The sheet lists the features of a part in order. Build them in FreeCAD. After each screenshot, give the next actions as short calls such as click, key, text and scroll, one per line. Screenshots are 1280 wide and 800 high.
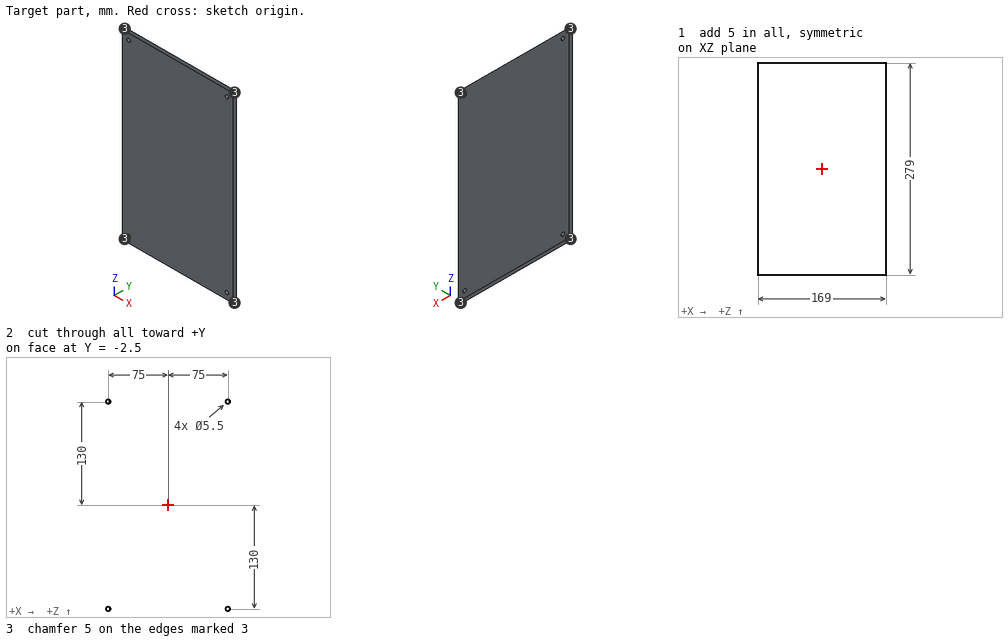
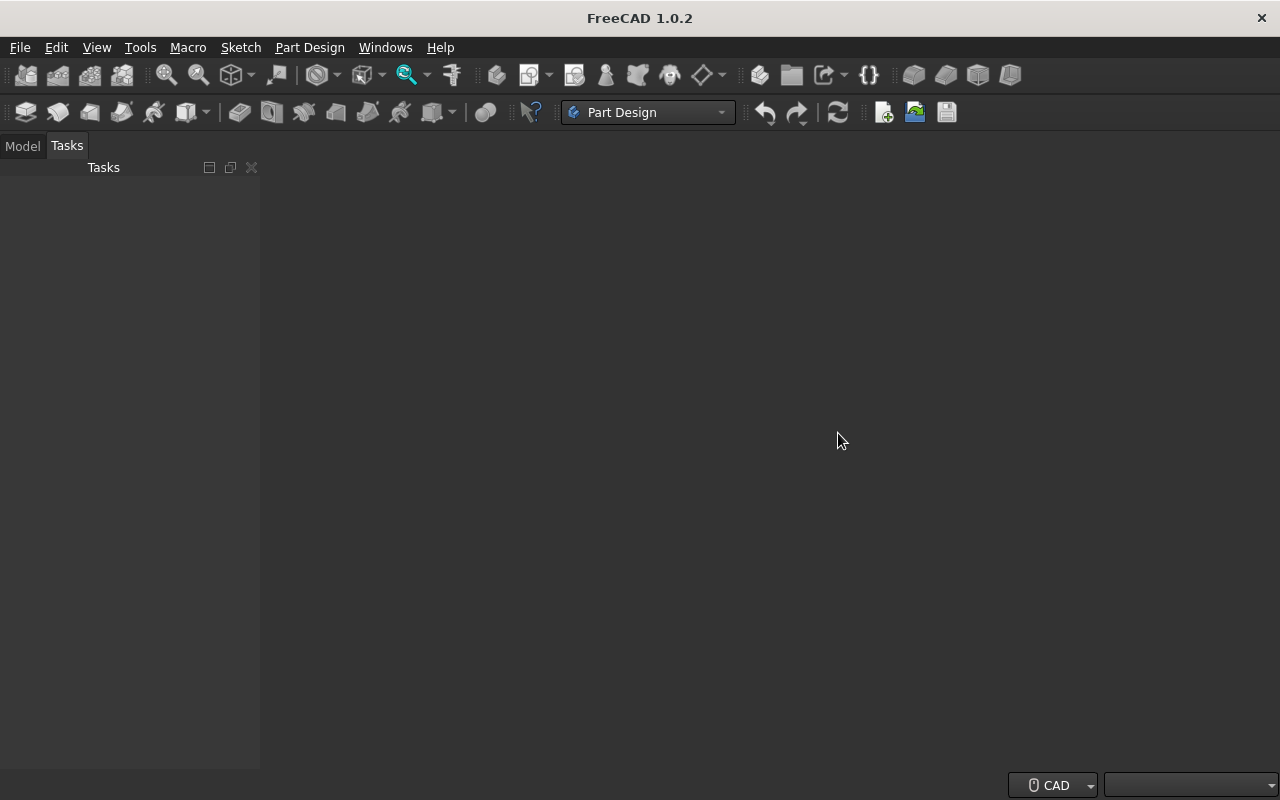
click(884, 112)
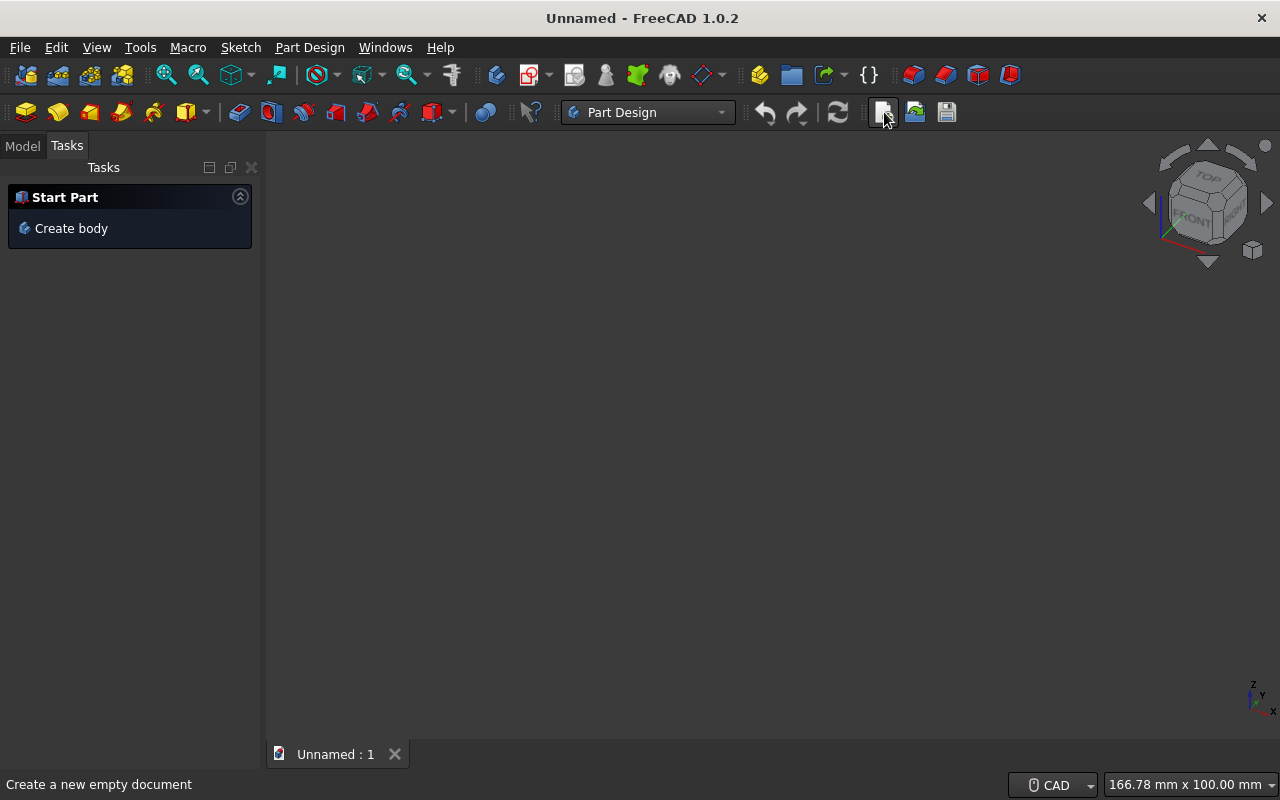
click(530, 76)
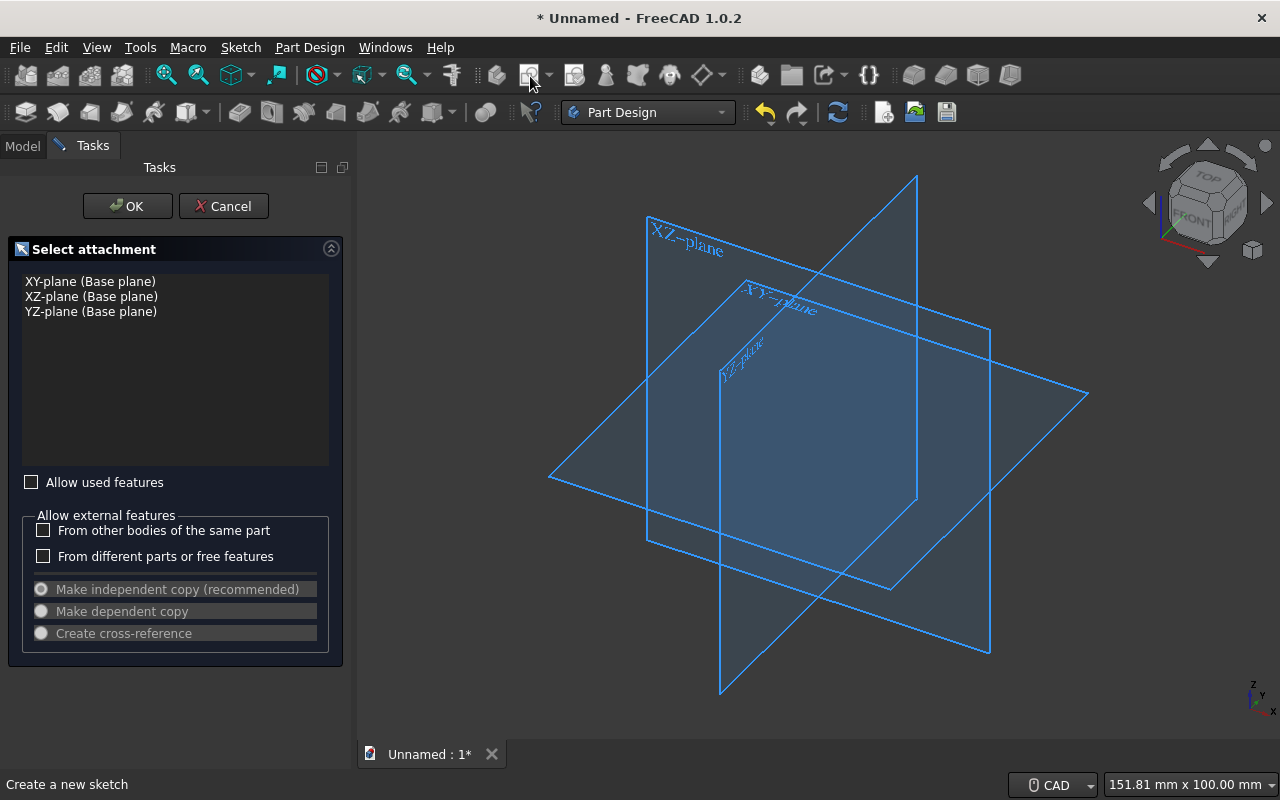
click(82, 296)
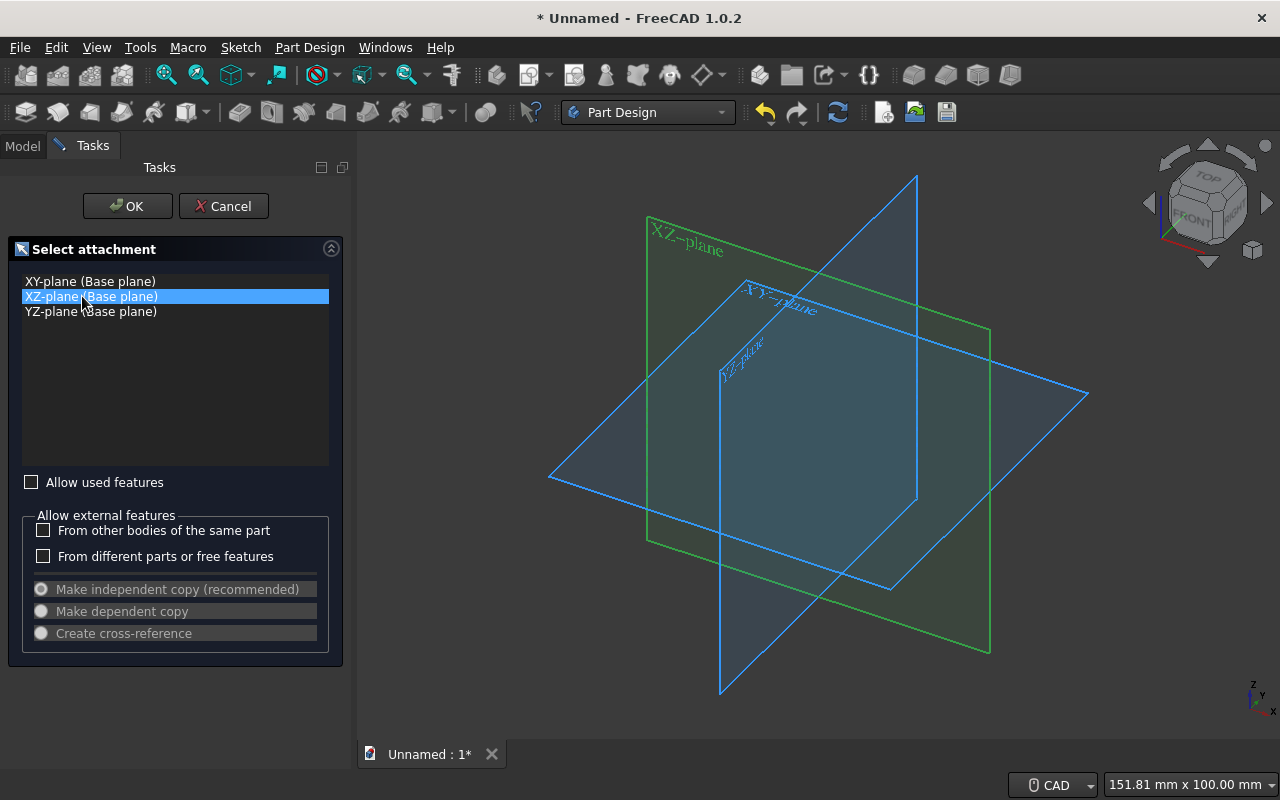
click(128, 206)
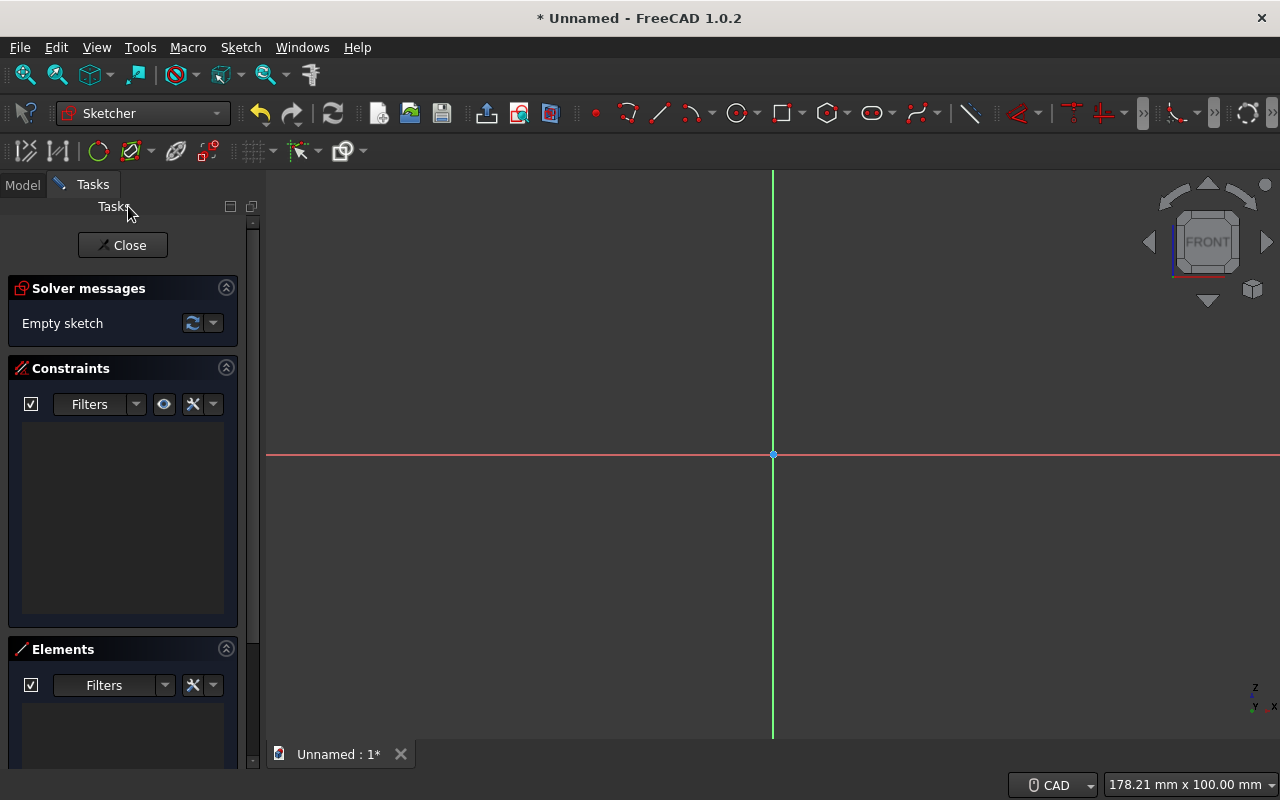
scroll(682, 454, down, 7)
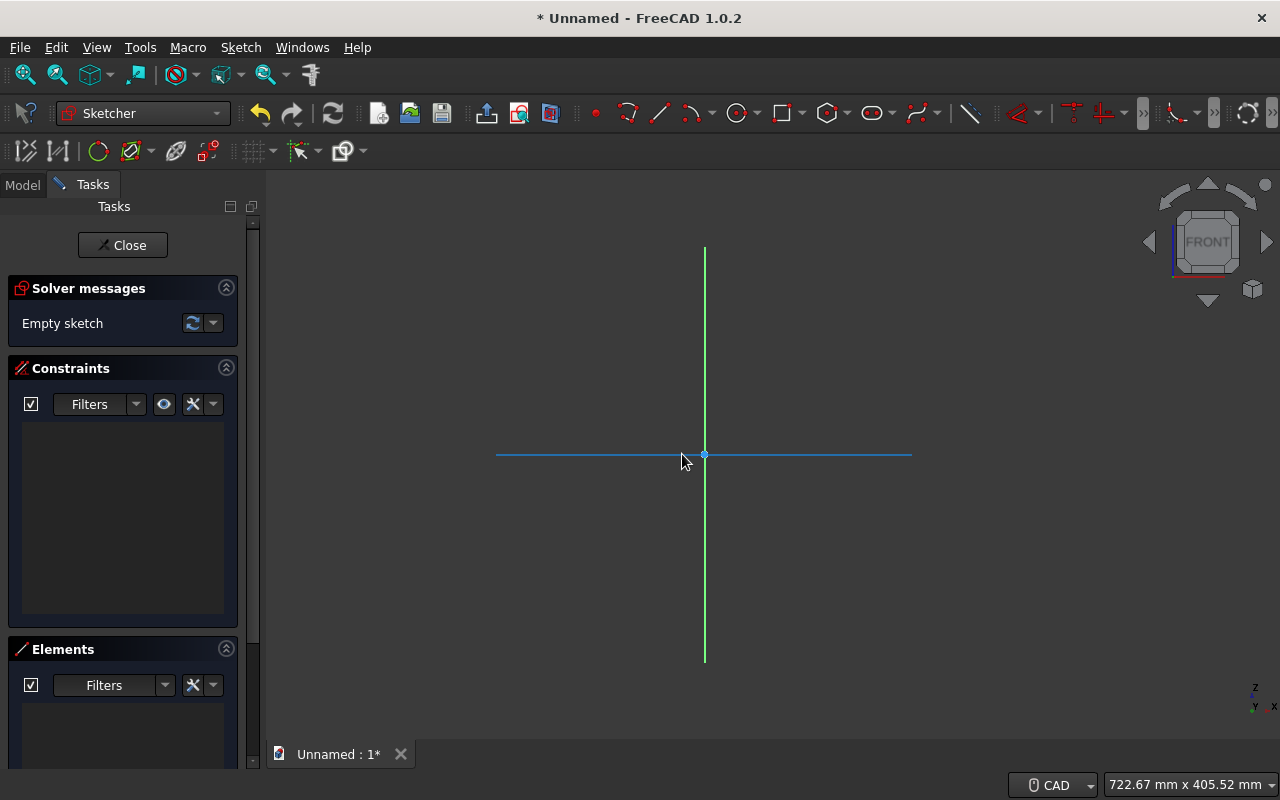
click(804, 114)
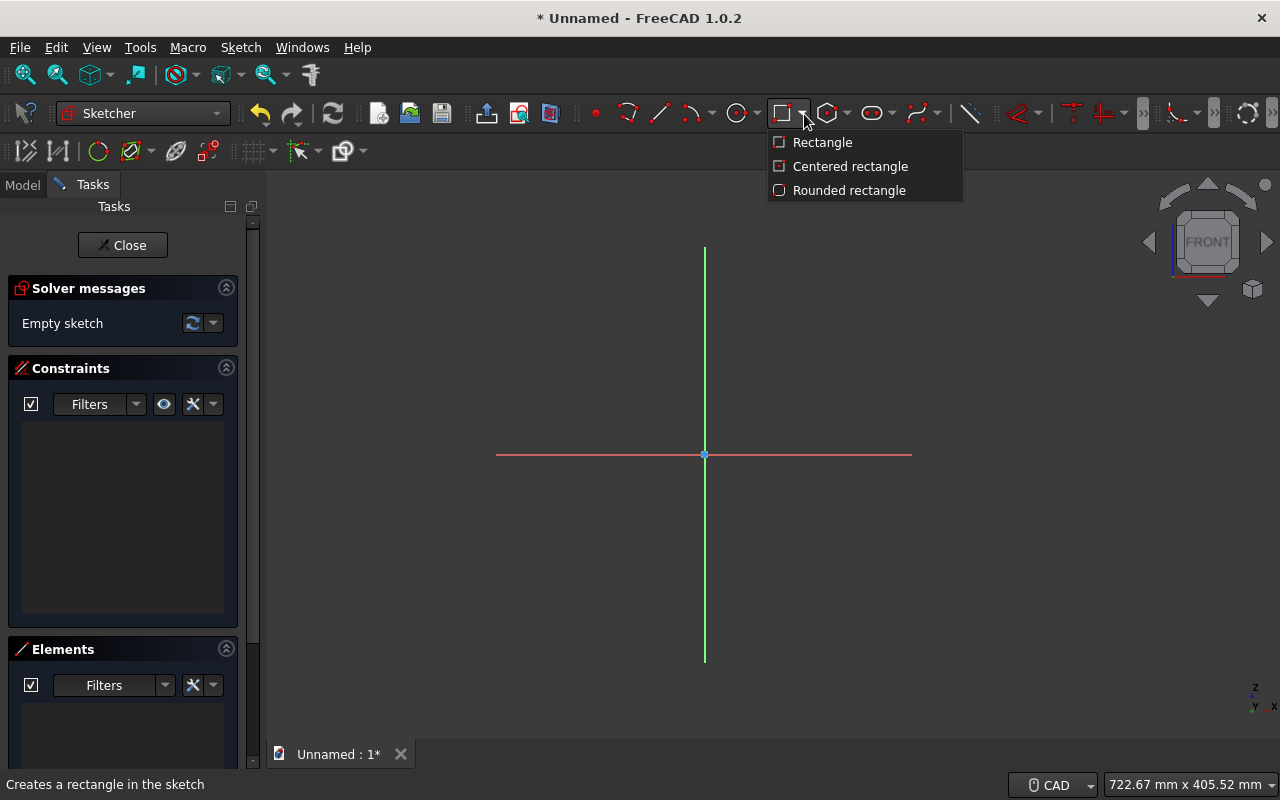
click(866, 166)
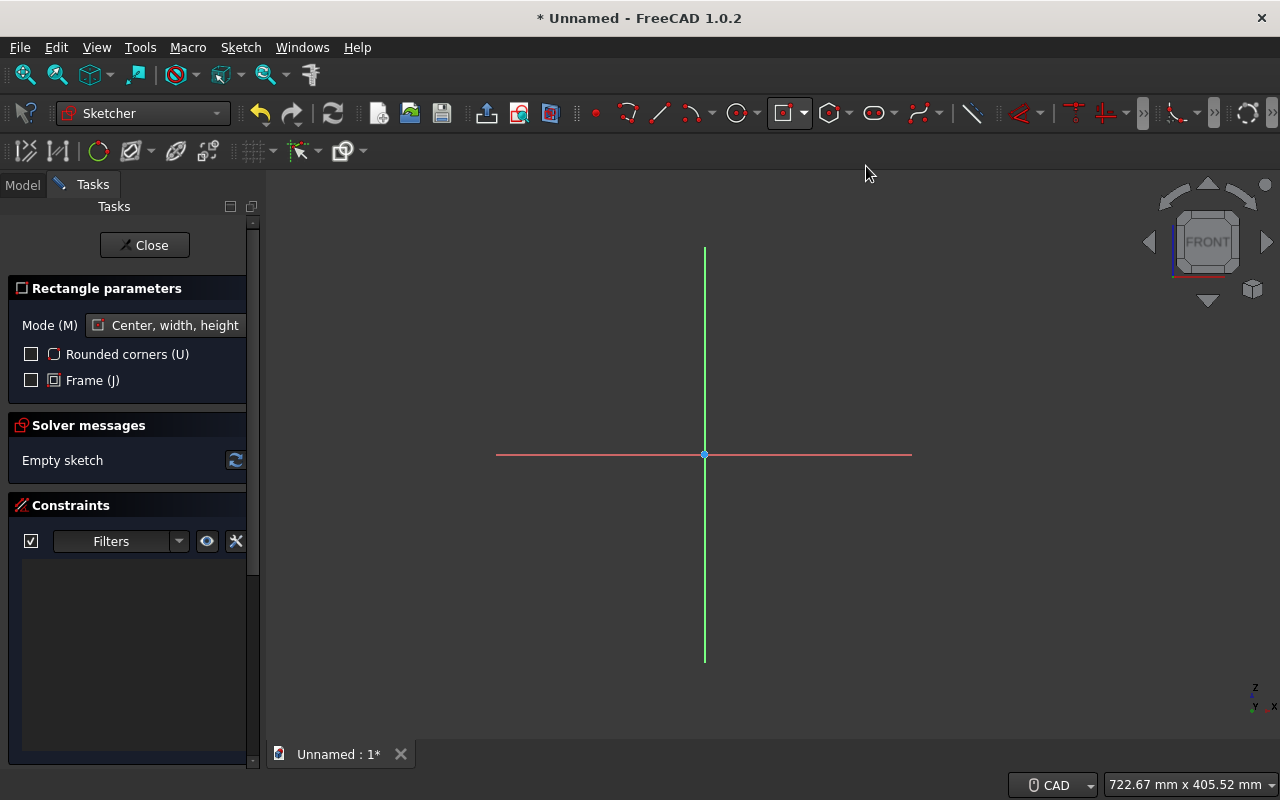
click(705, 454)
click(823, 259)
key(Escape)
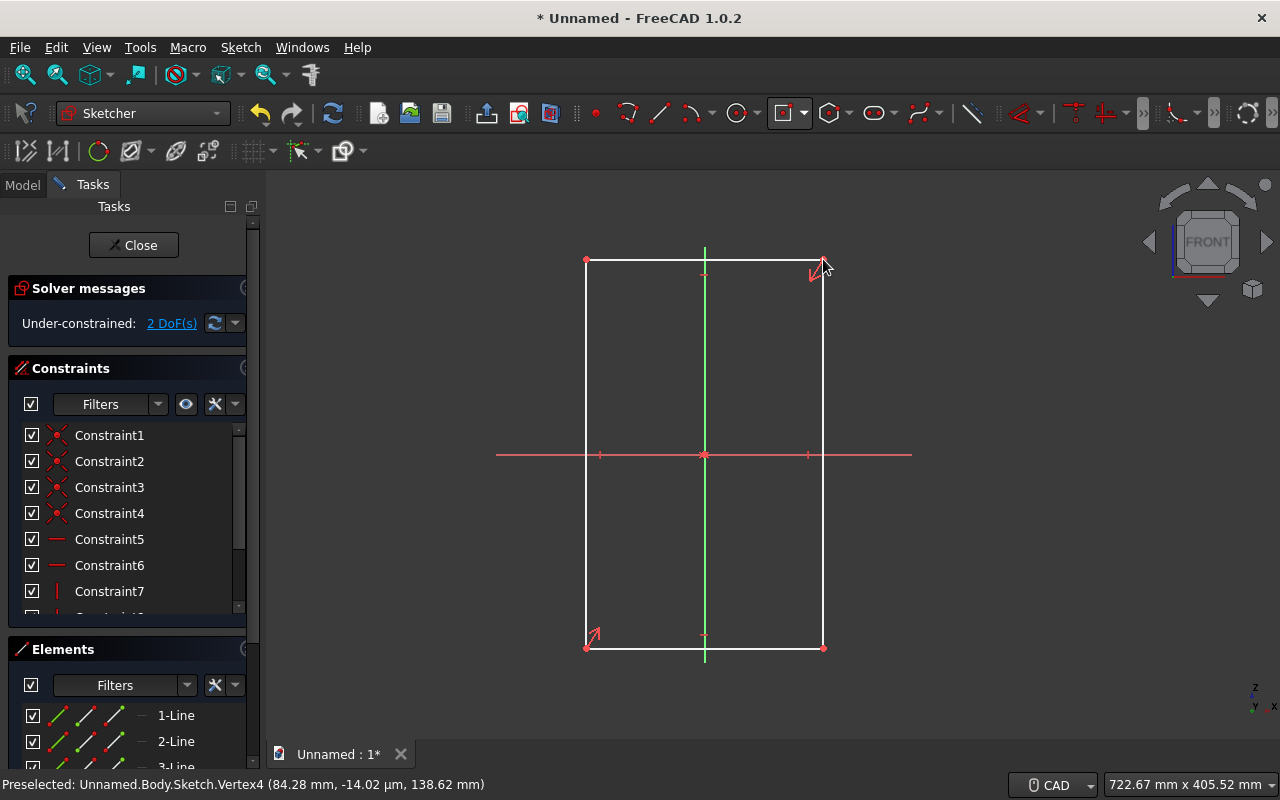
click(1020, 114)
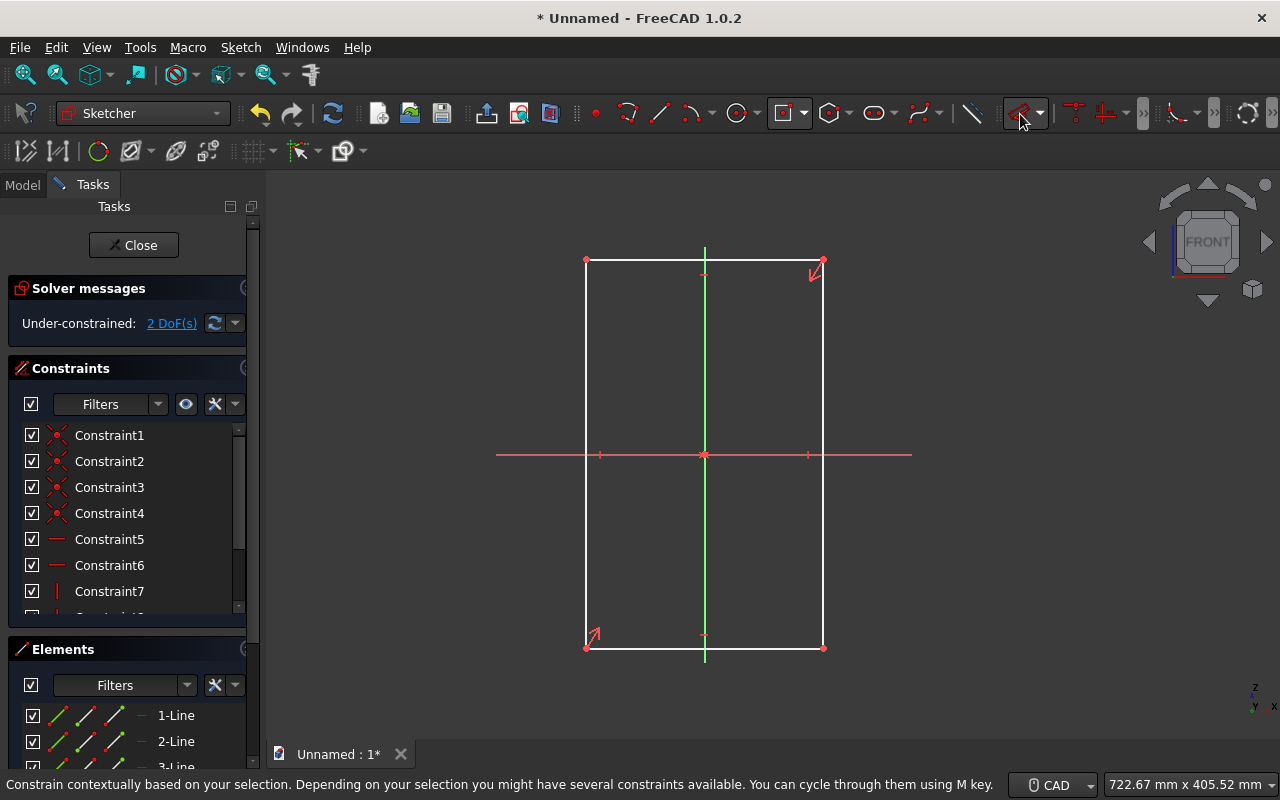
click(657, 649)
click(650, 683)